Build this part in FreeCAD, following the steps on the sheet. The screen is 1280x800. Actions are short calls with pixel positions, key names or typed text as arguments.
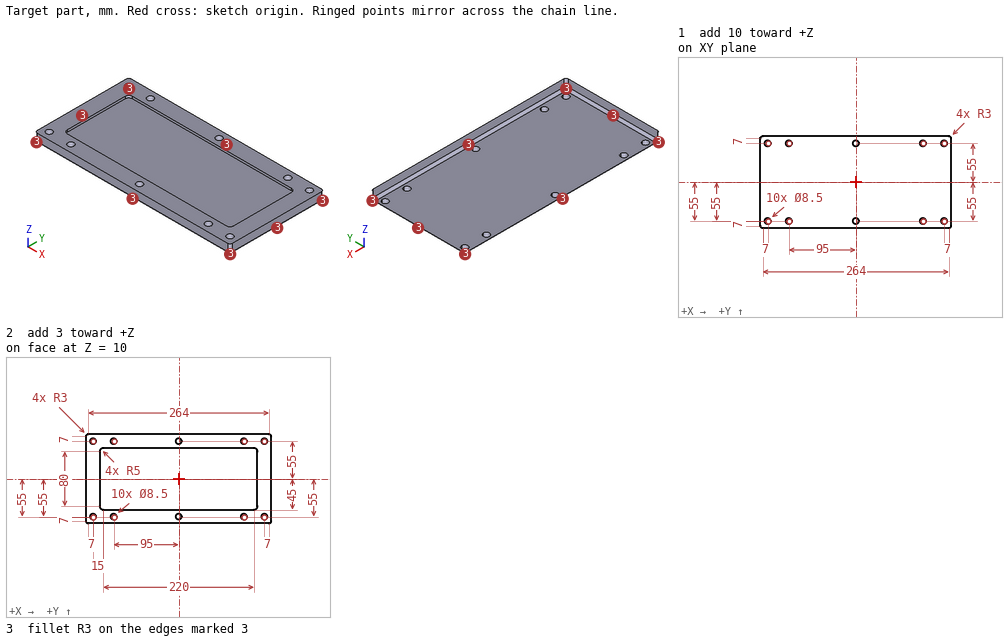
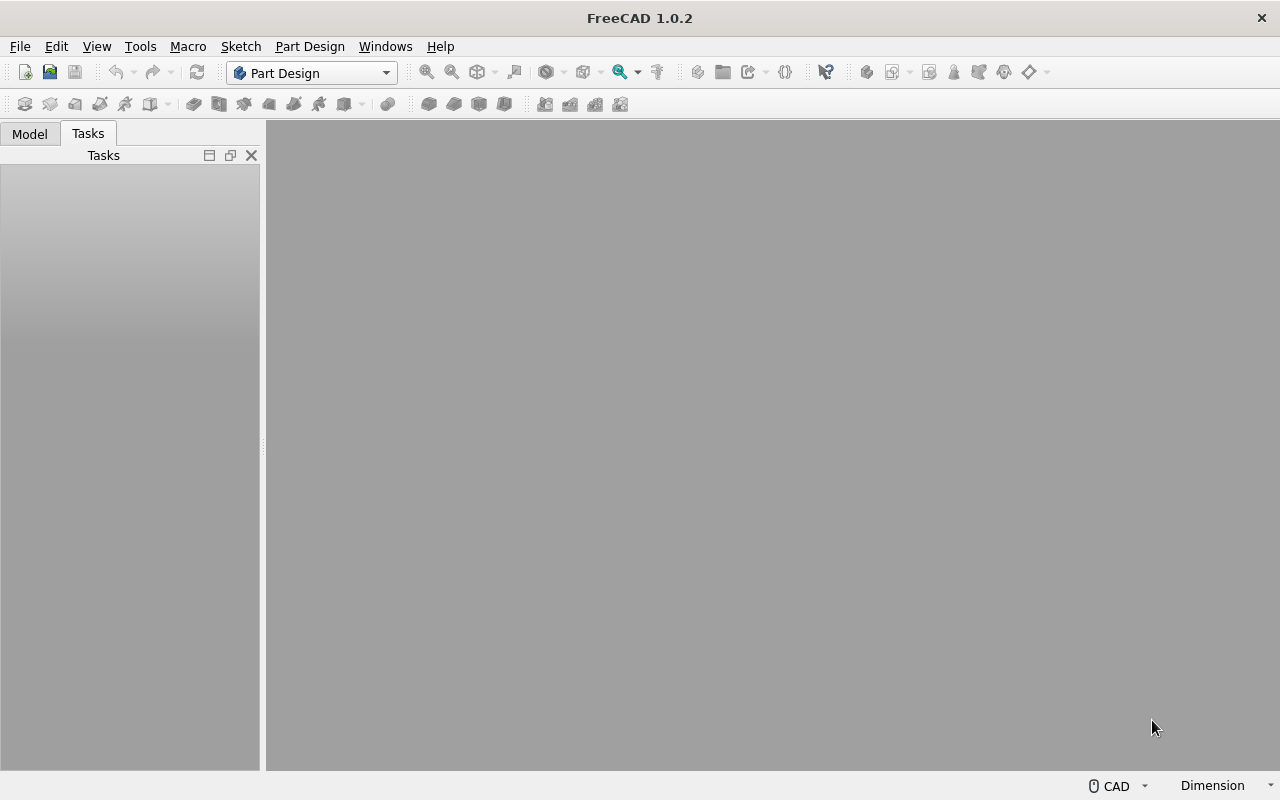
click(25, 72)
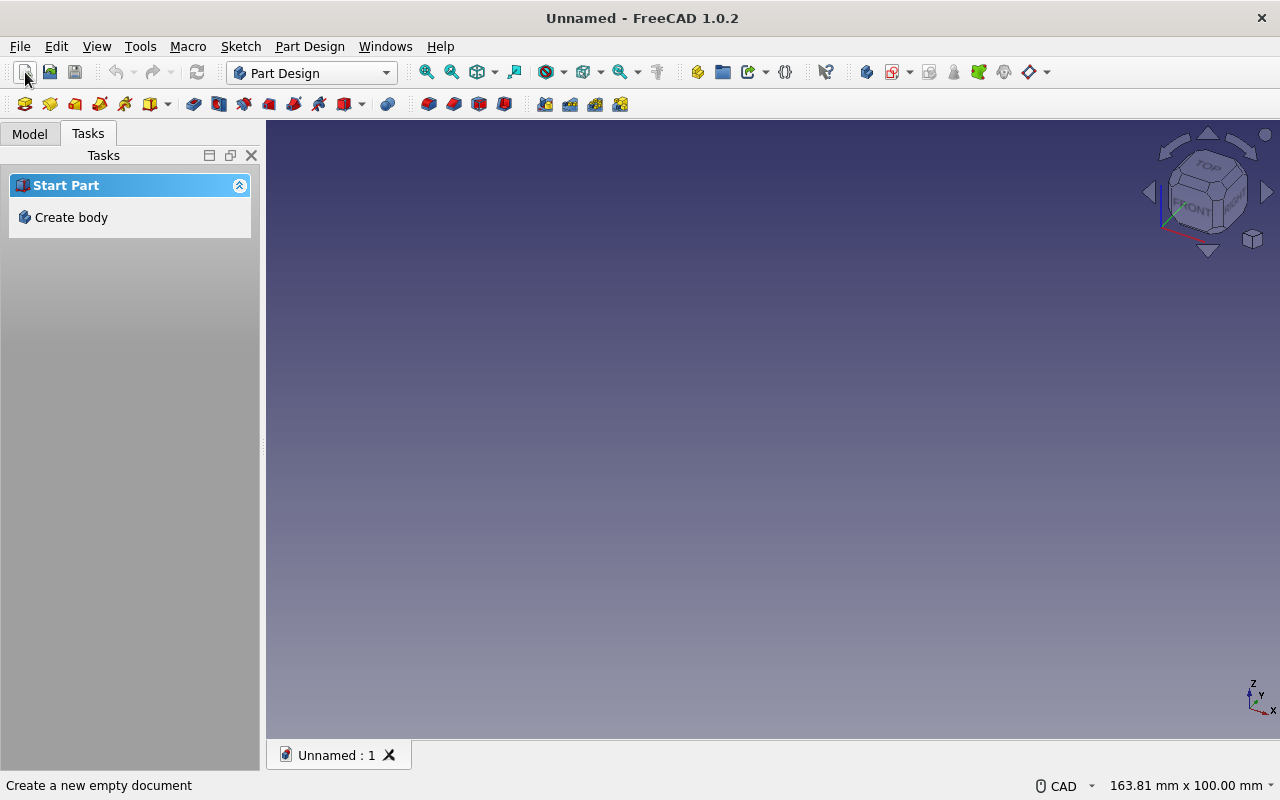
click(892, 72)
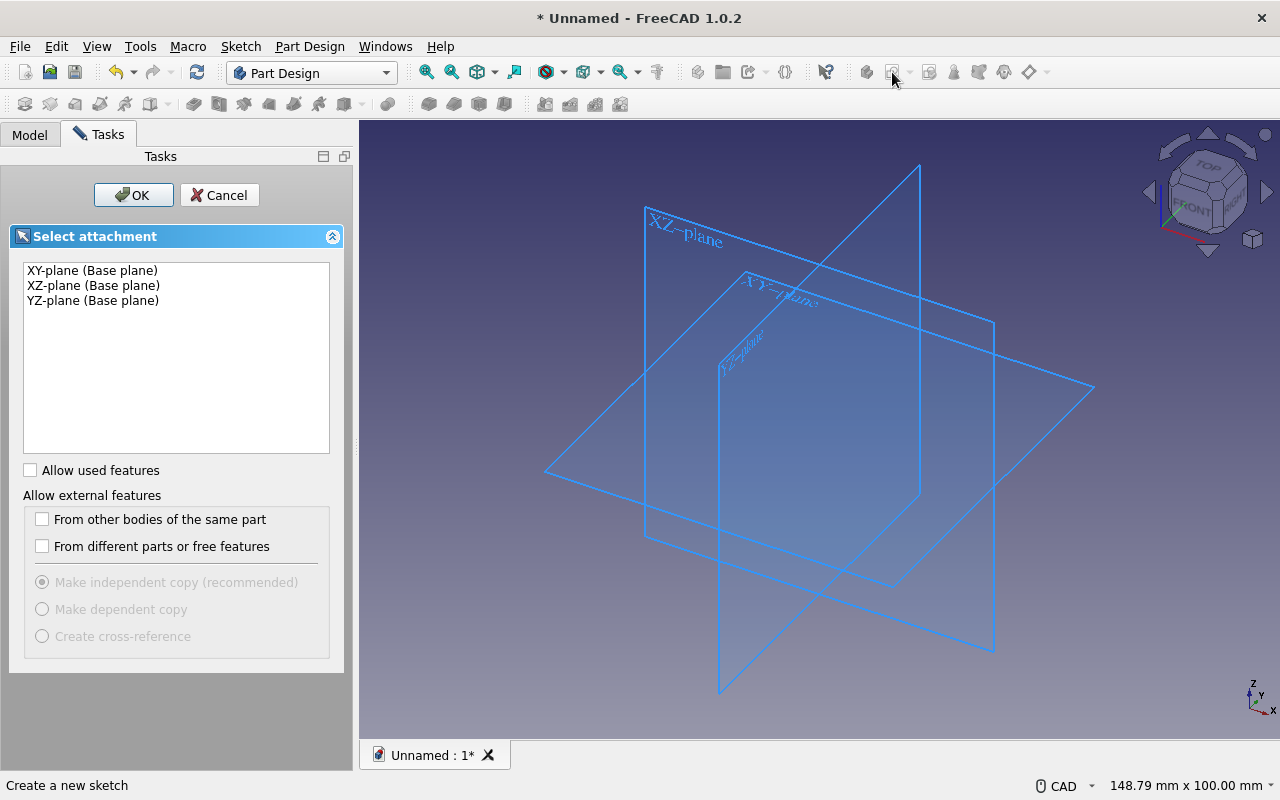
click(84, 270)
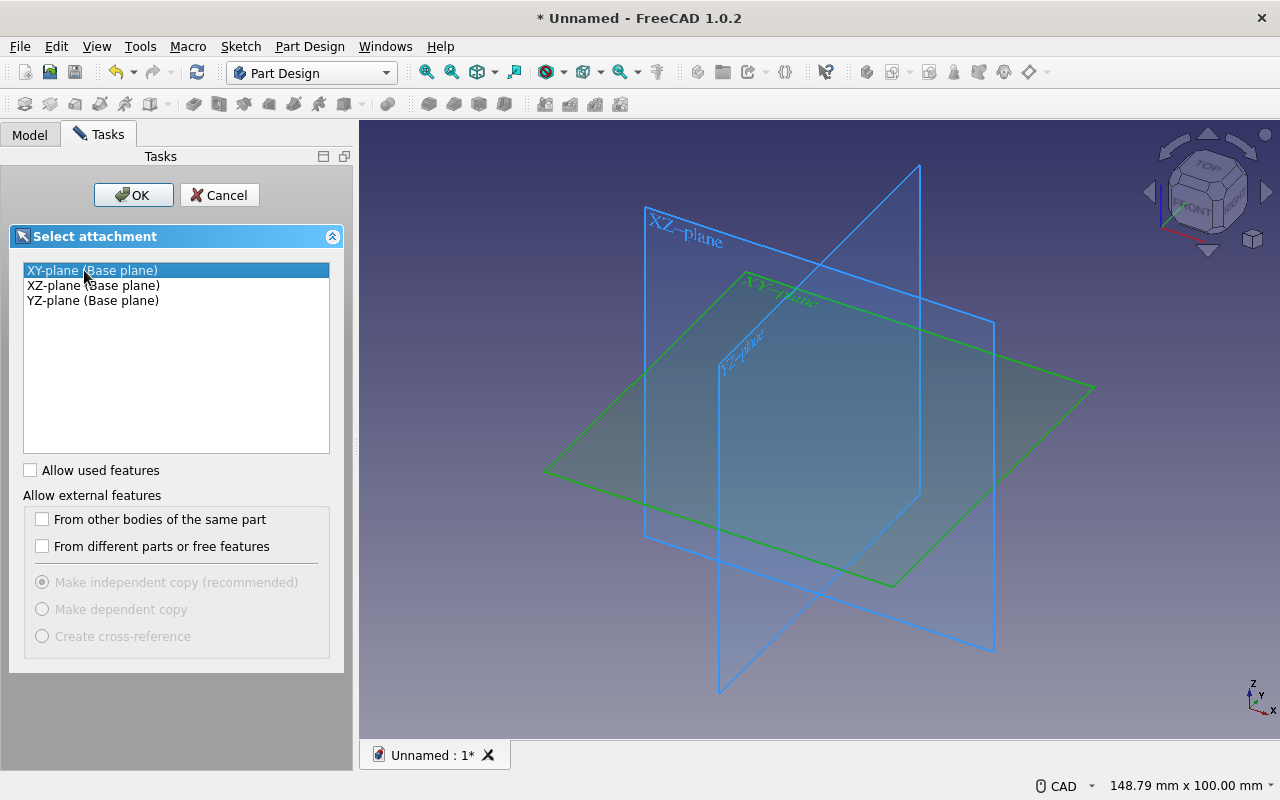
click(134, 195)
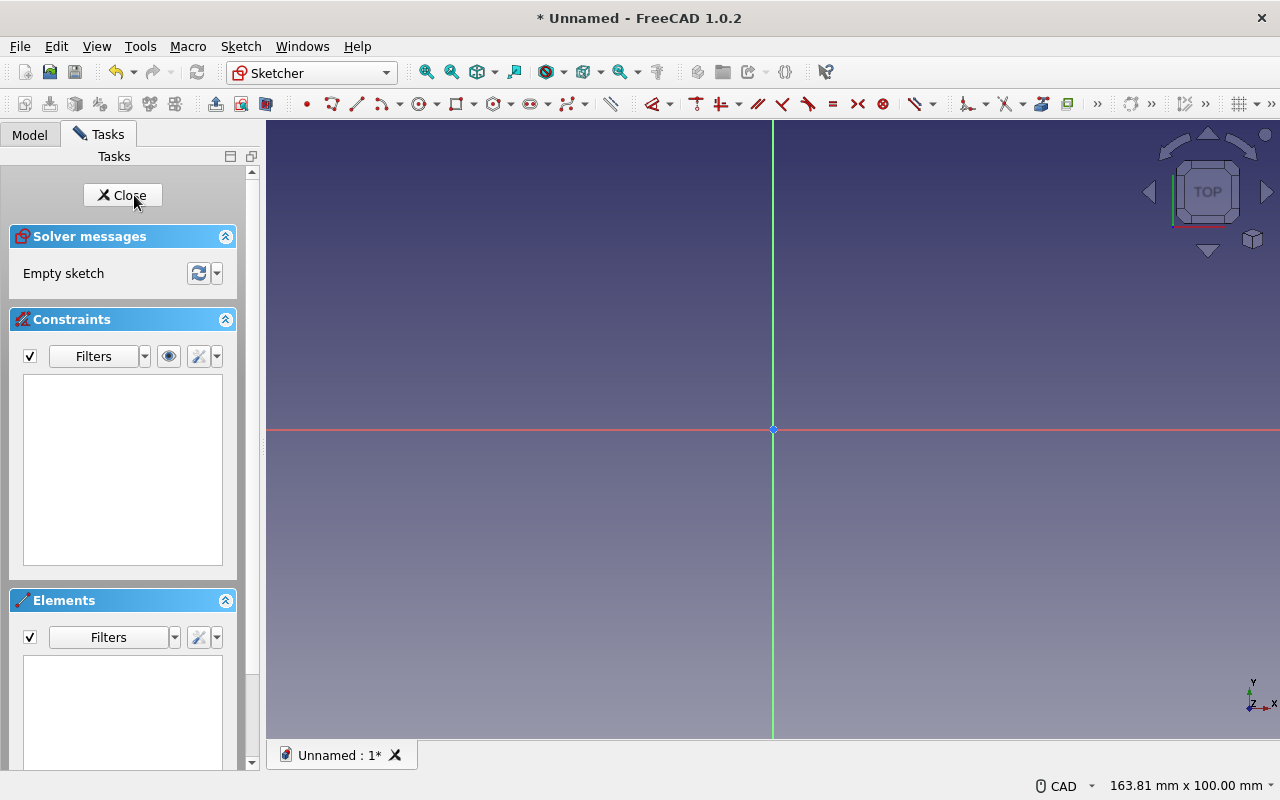
scroll(665, 430, down, 5)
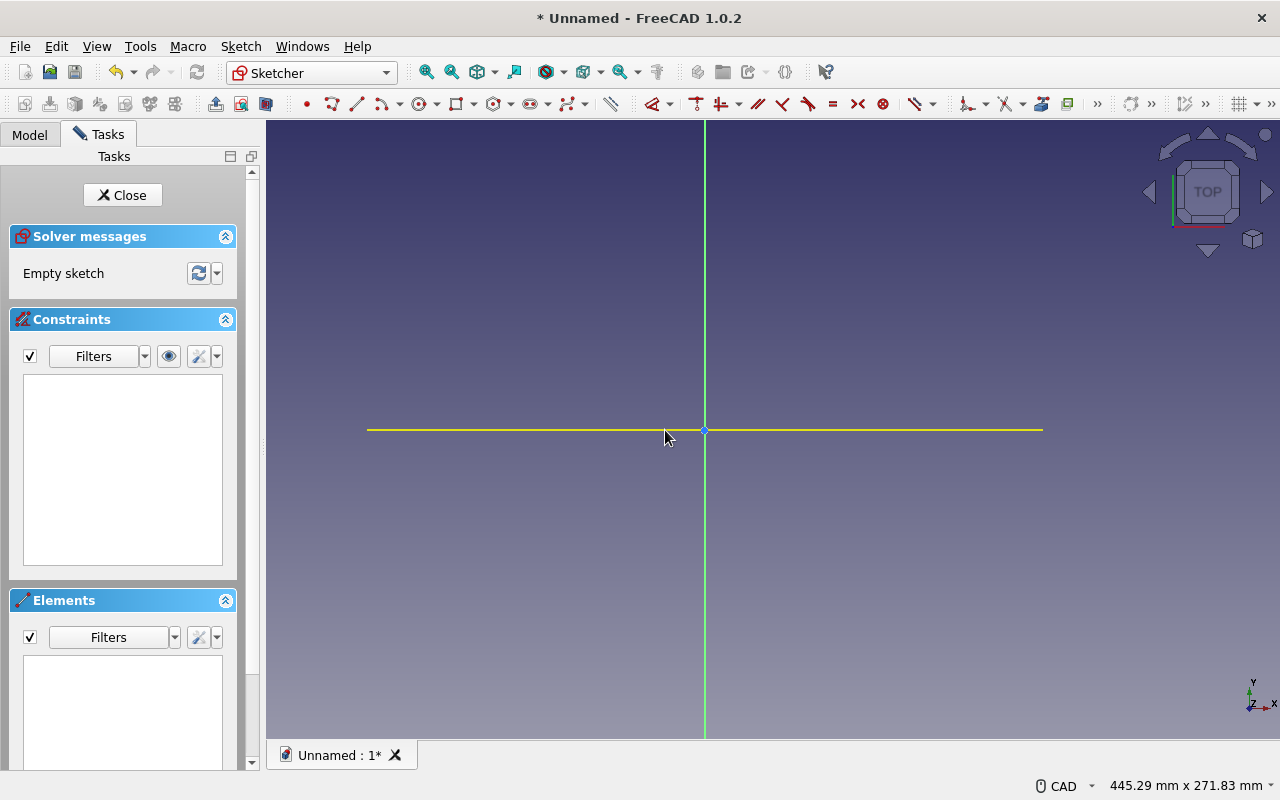
click(357, 104)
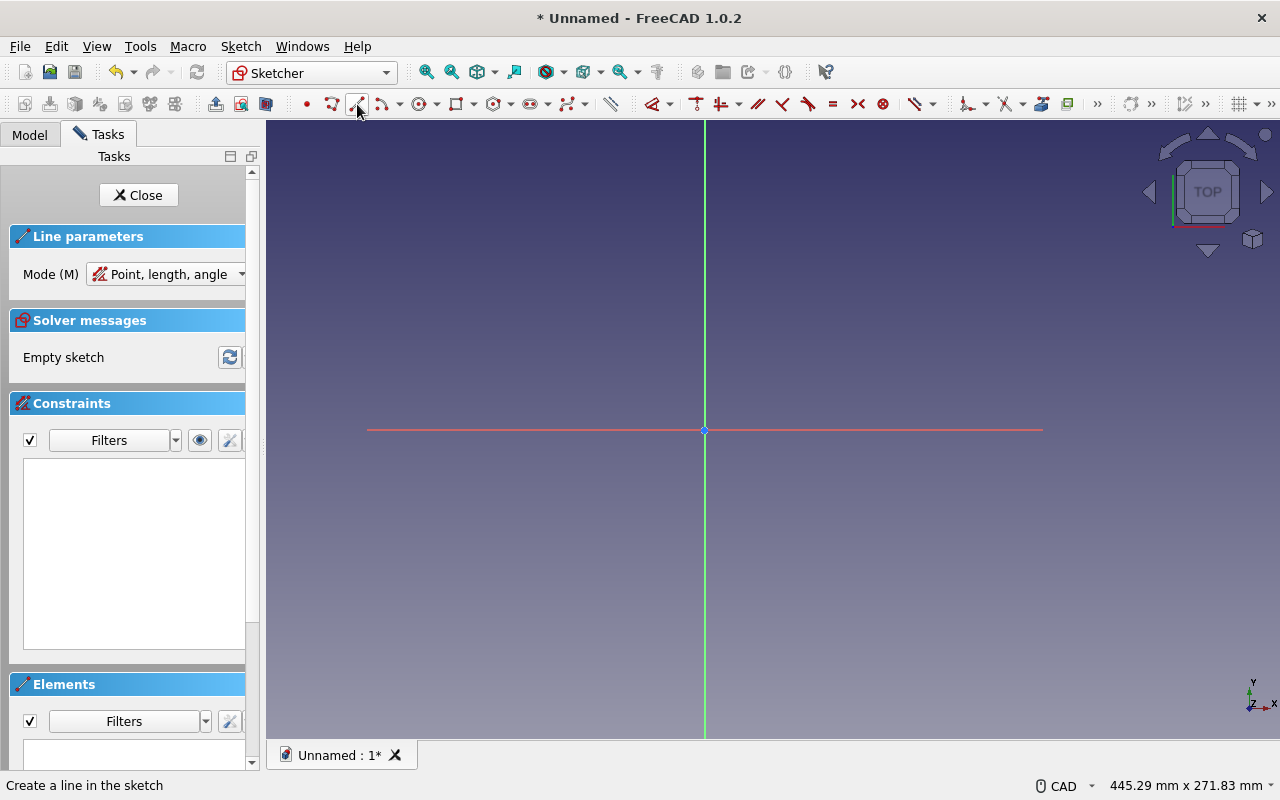
click(404, 578)
click(1006, 578)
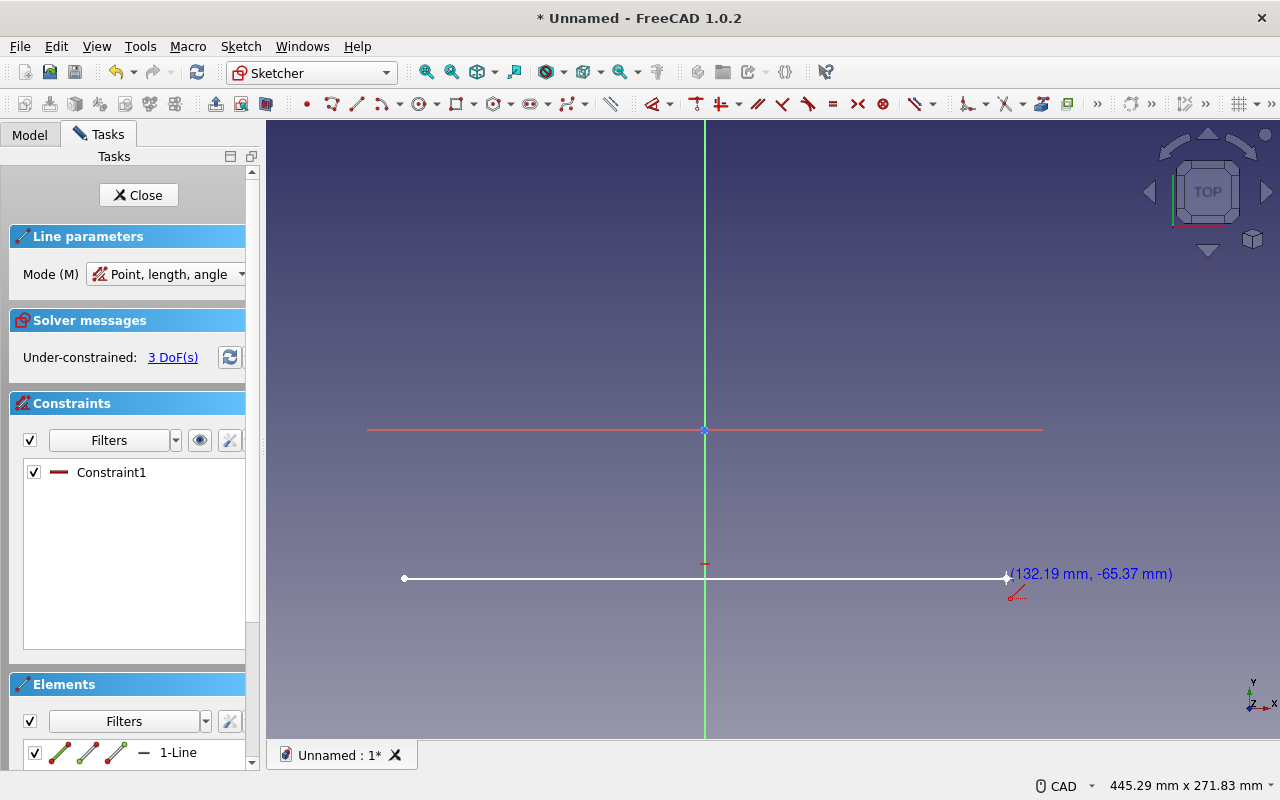
scroll(1012, 571, up, 3)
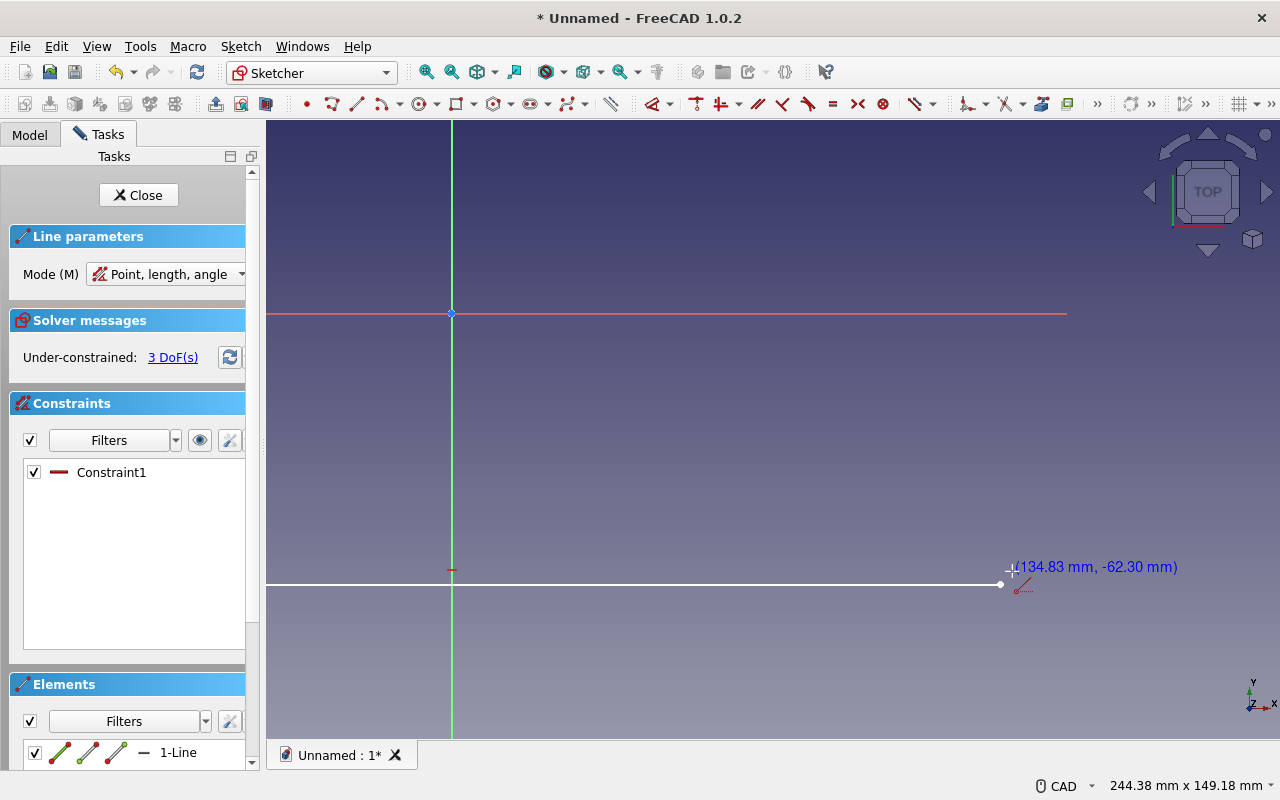
click(1012, 571)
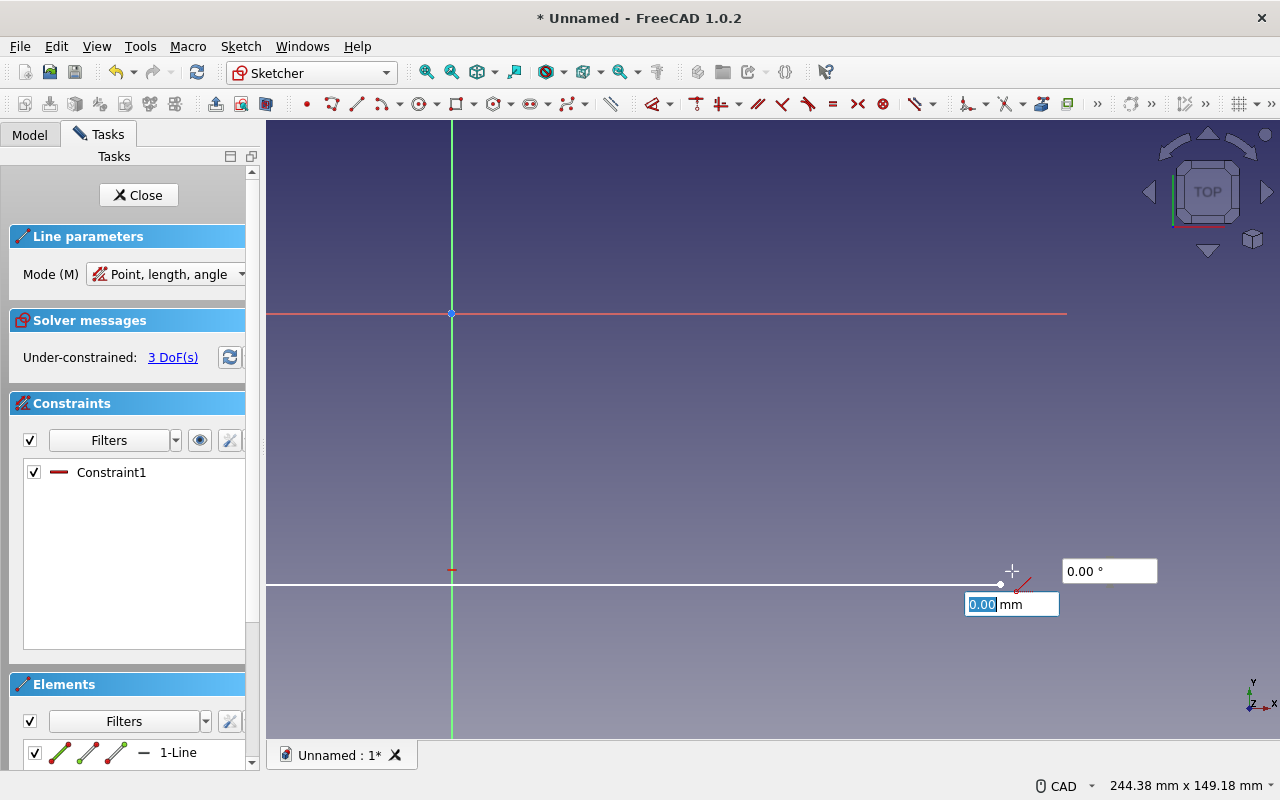
scroll(1012, 570, down, 3)